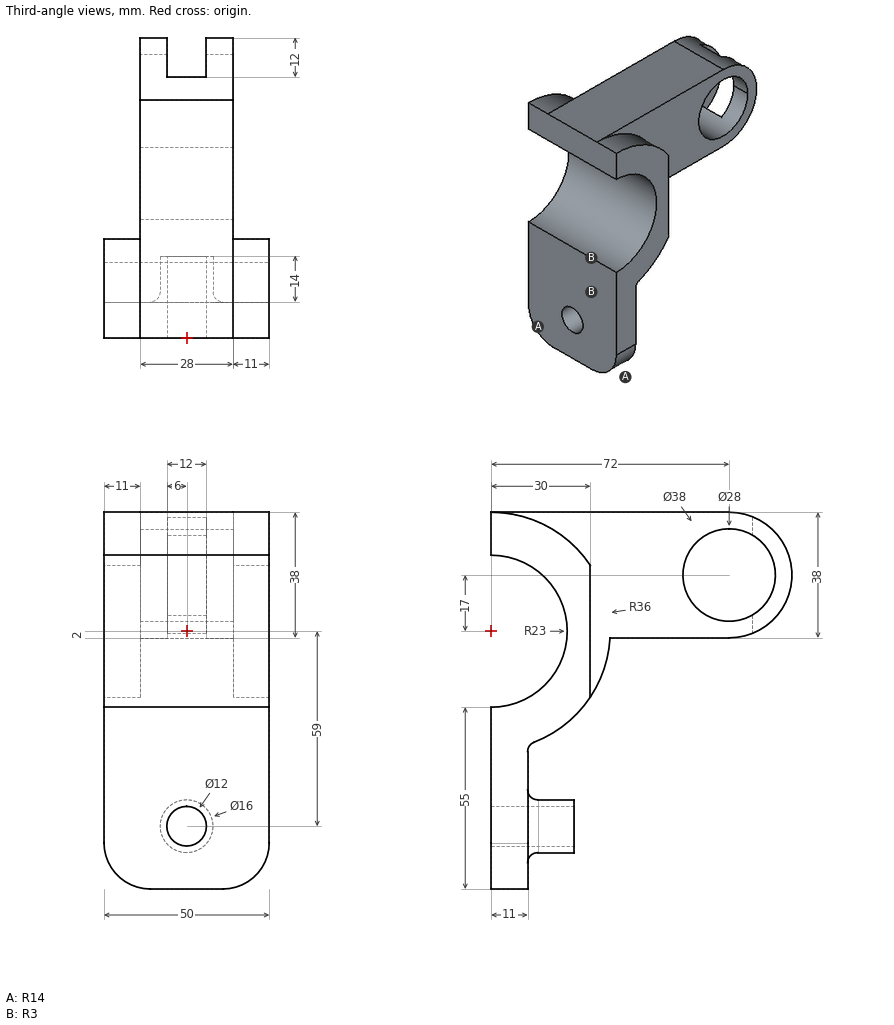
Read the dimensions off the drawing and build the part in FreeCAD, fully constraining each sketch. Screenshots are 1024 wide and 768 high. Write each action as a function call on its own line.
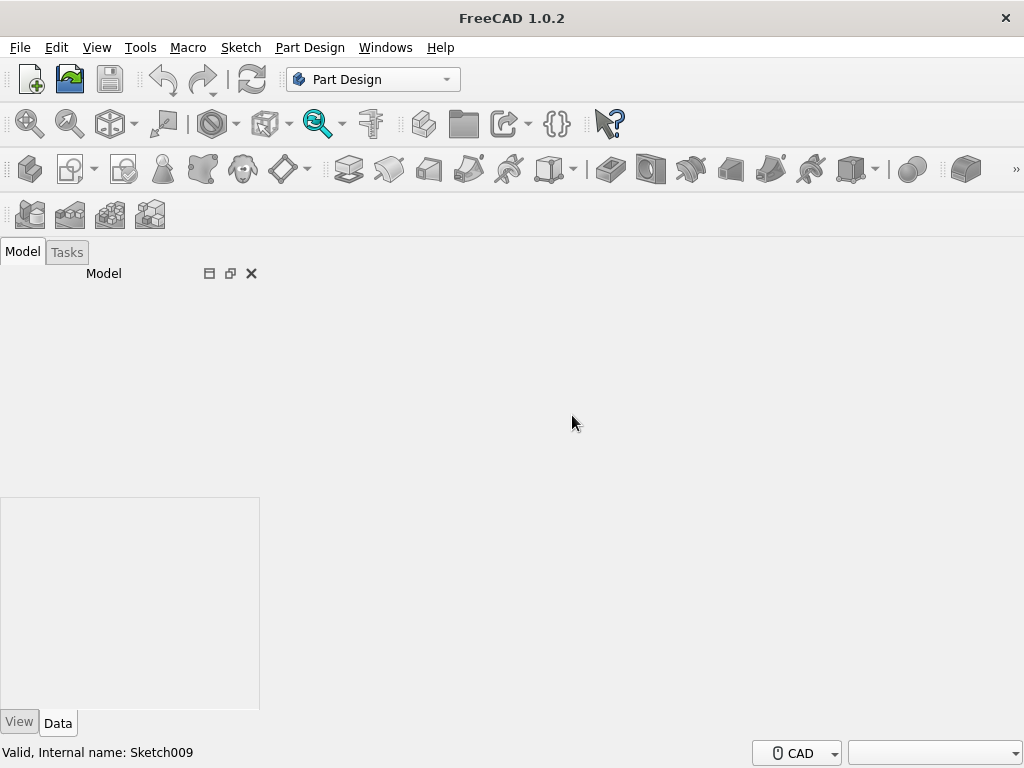
click(30, 80)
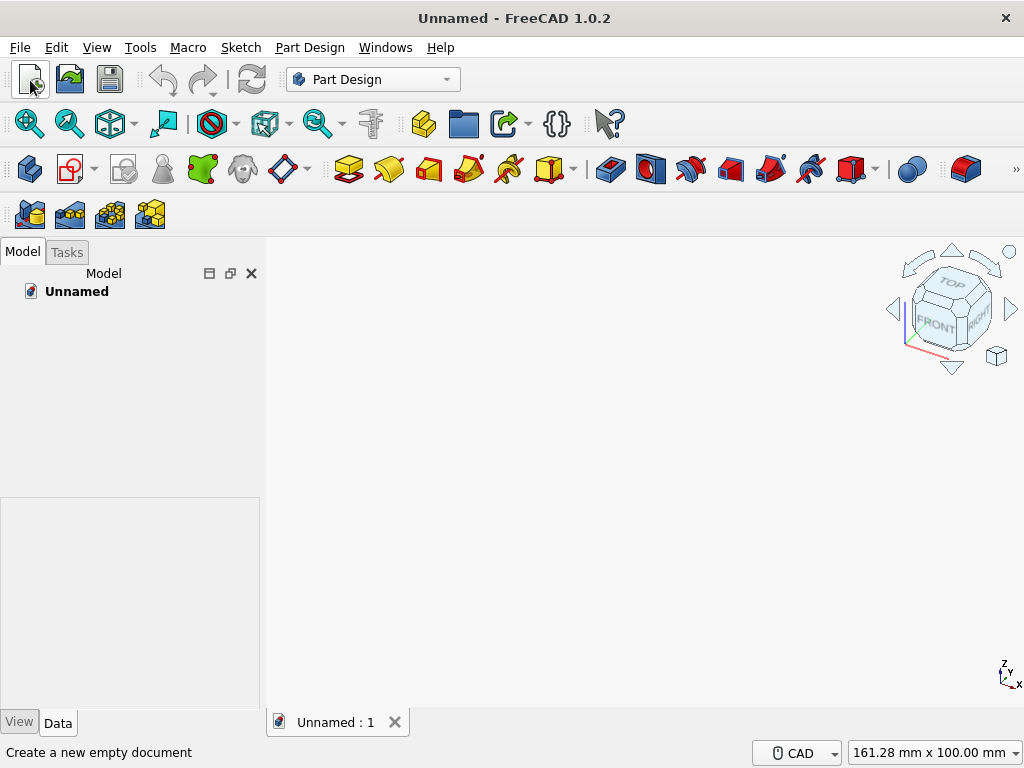
click(70, 170)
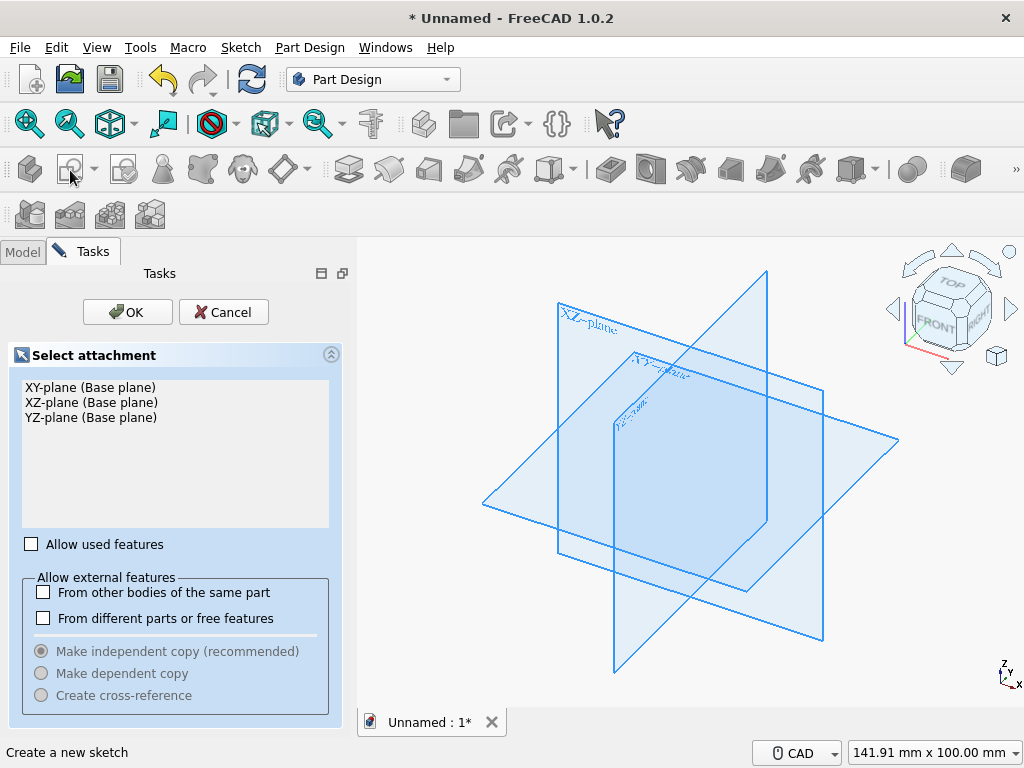
click(82, 418)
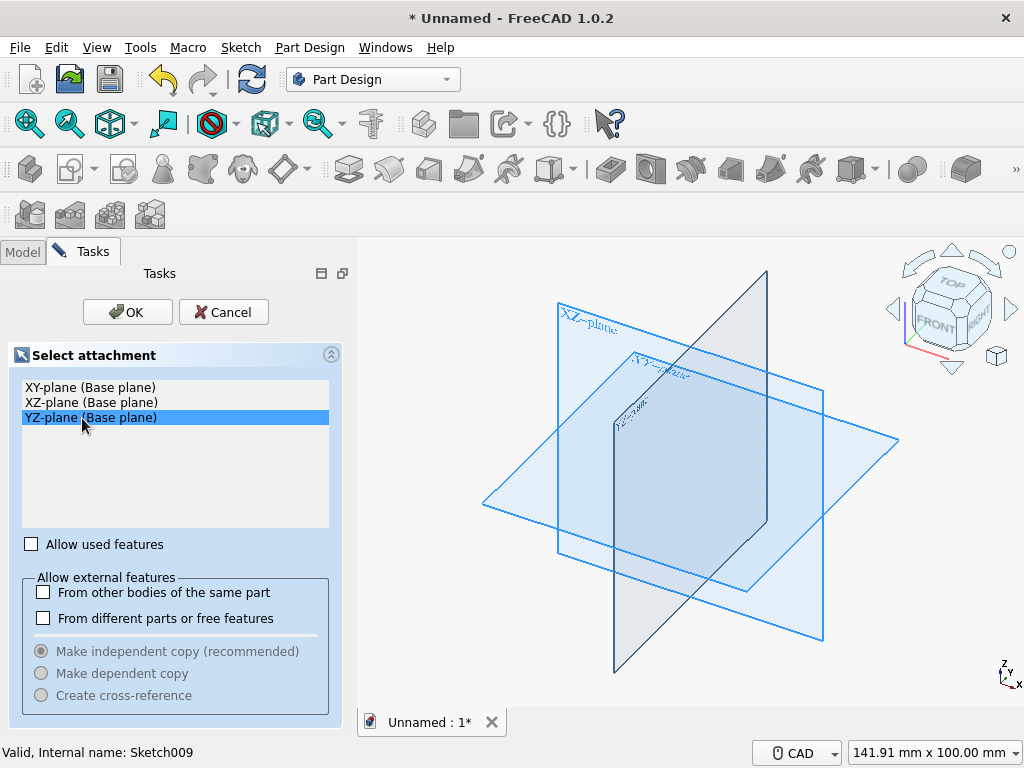
click(128, 312)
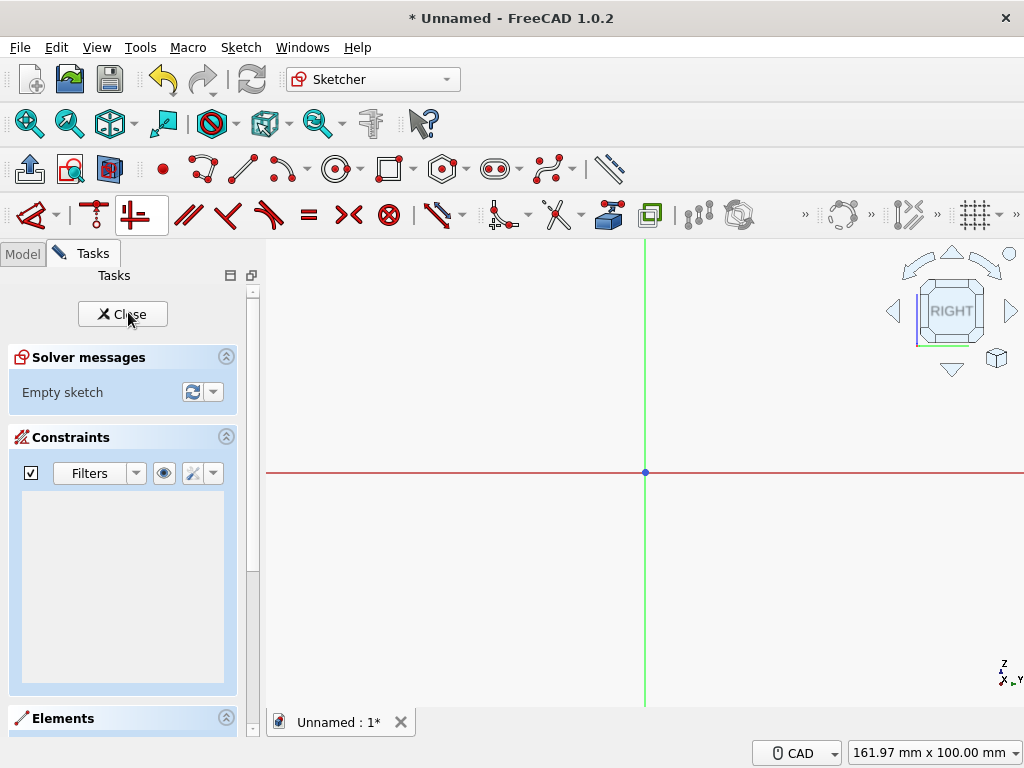
scroll(392, 353, down, 3)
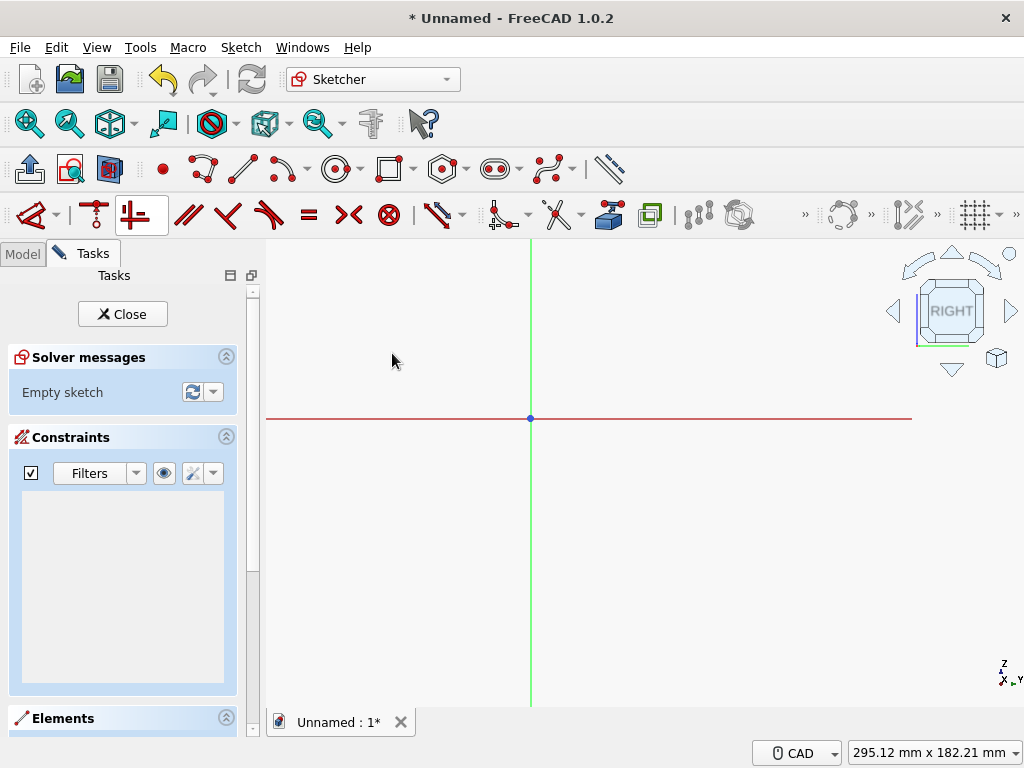
click(204, 170)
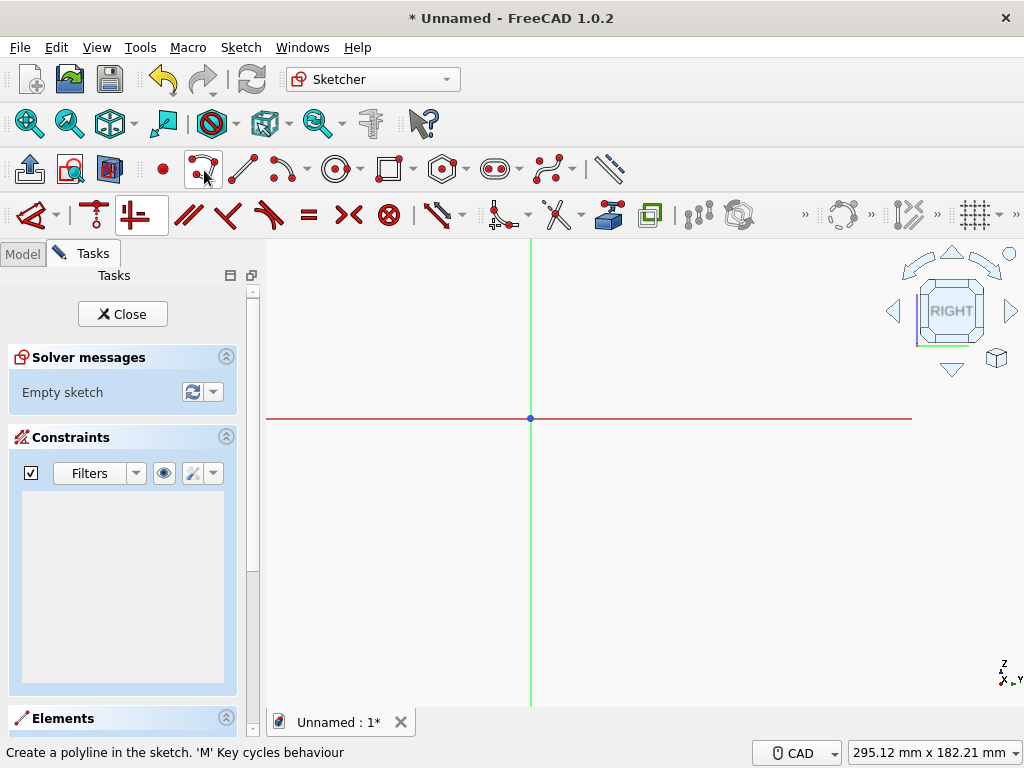
click(531, 478)
click(540, 619)
click(559, 619)
click(559, 507)
right_click(559, 507)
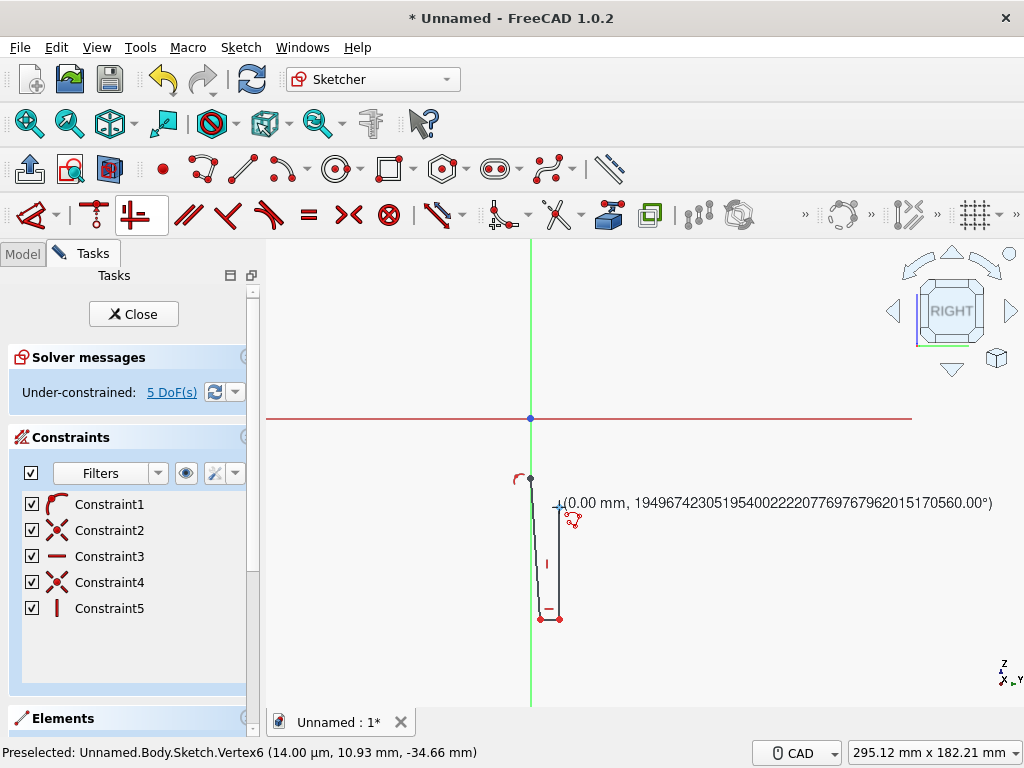
click(244, 170)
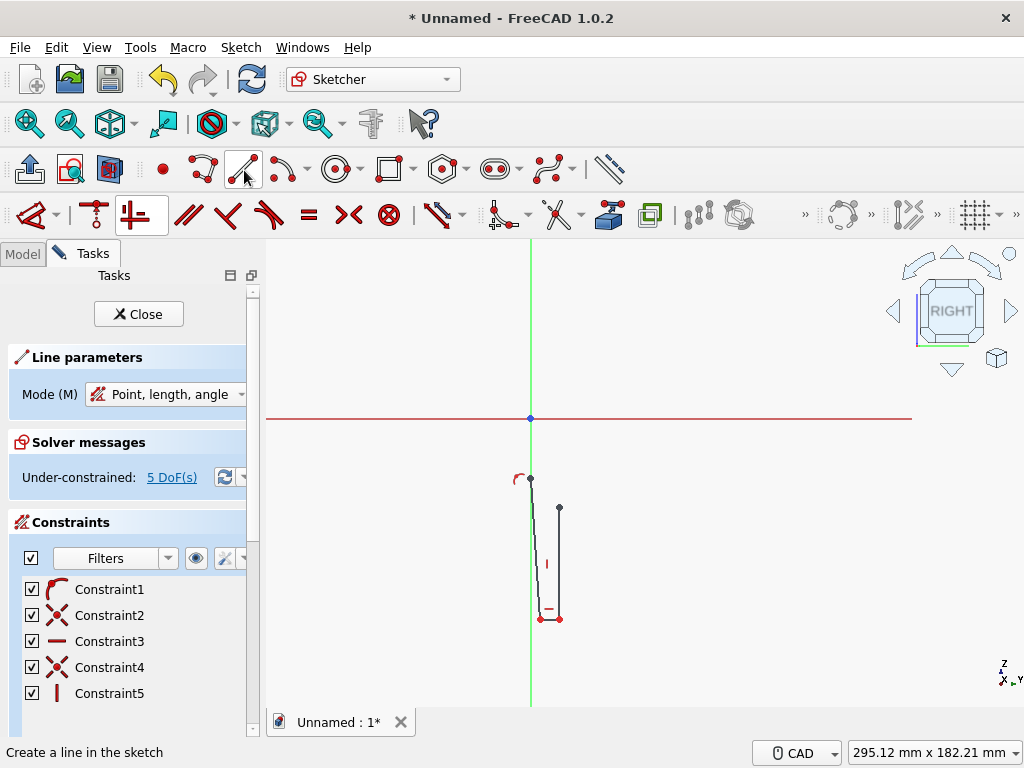
click(531, 327)
click(540, 360)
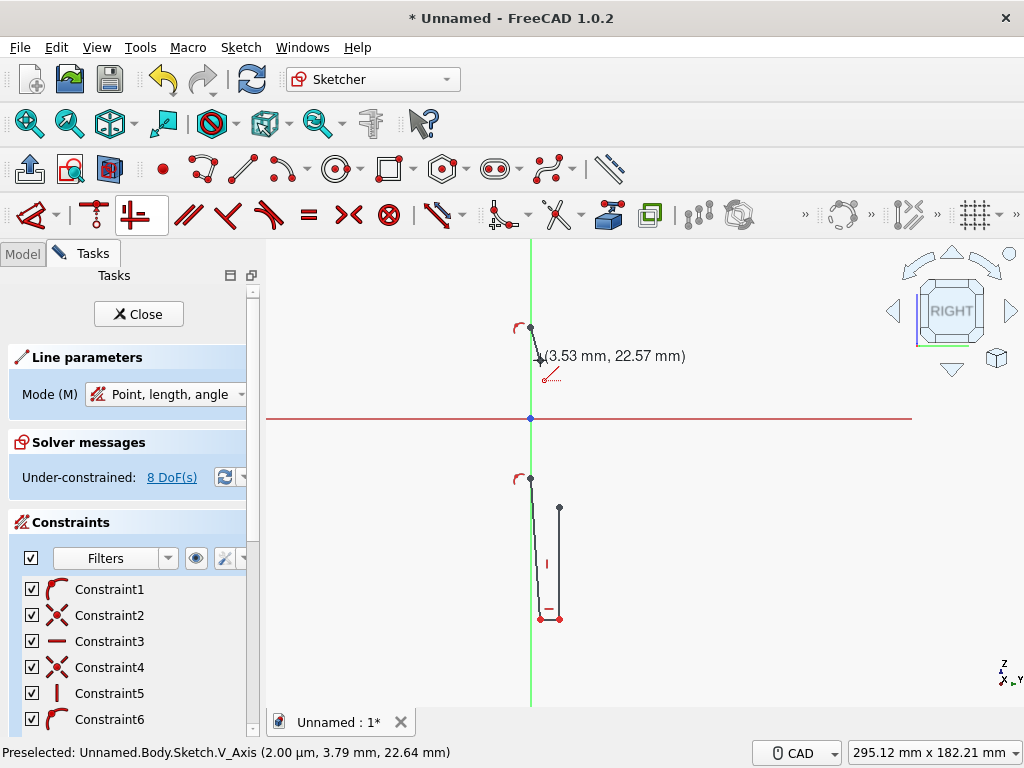
click(310, 170)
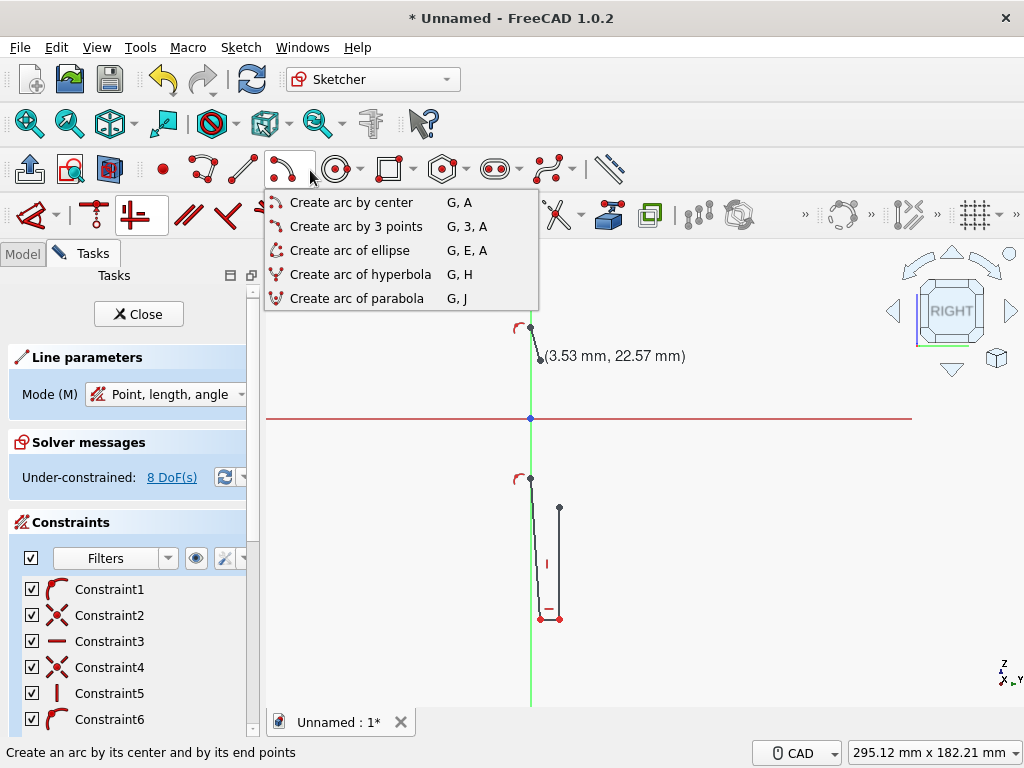
click(402, 226)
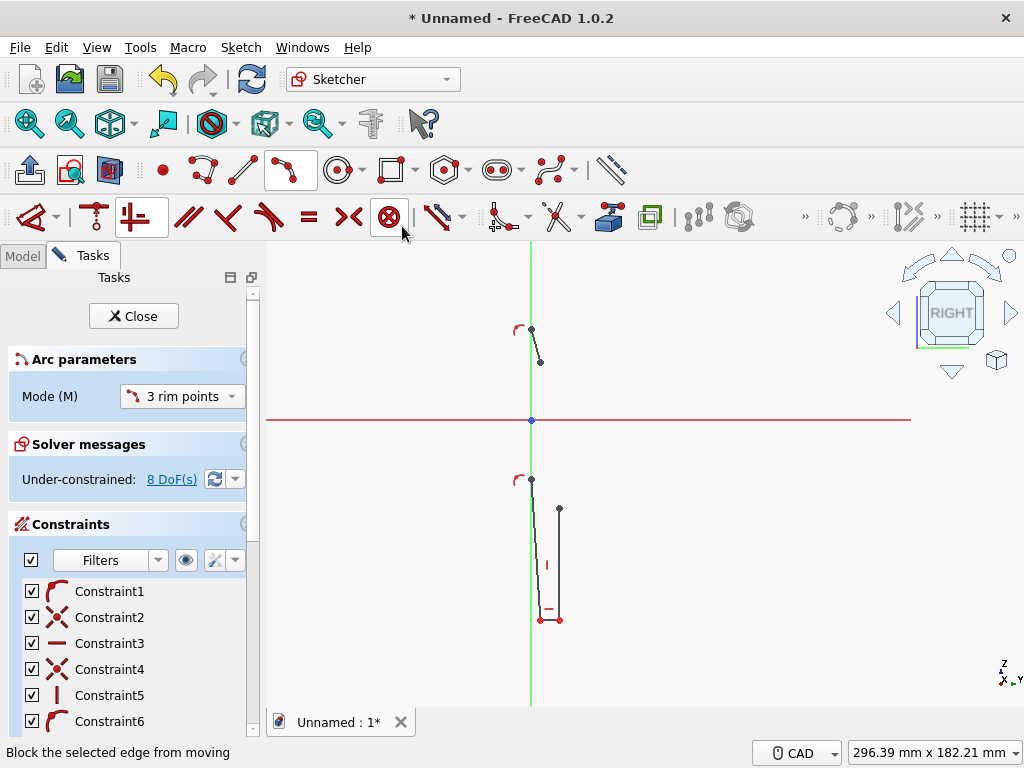
click(559, 509)
click(531, 330)
click(622, 406)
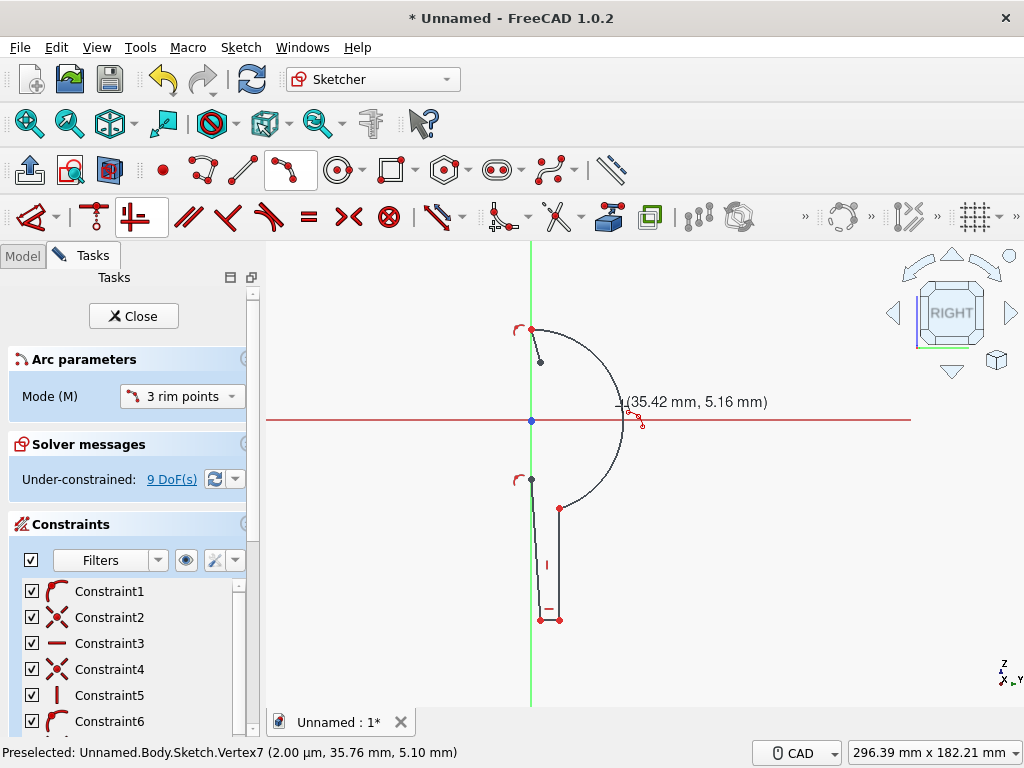
click(540, 362)
click(531, 480)
click(587, 438)
key(Escape)